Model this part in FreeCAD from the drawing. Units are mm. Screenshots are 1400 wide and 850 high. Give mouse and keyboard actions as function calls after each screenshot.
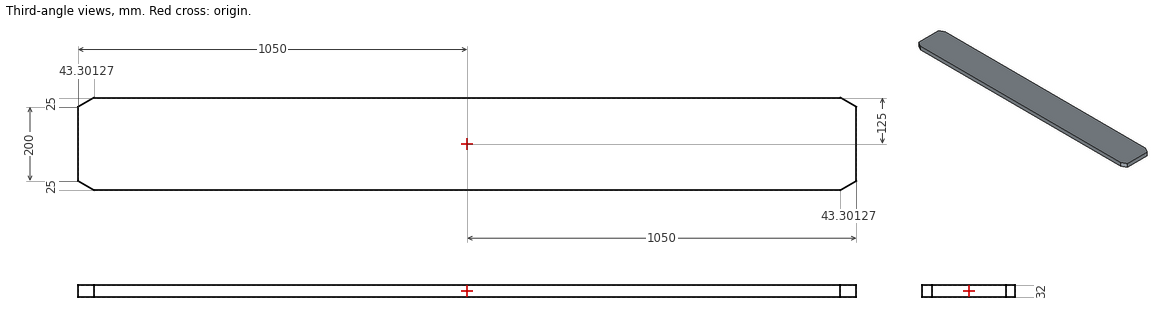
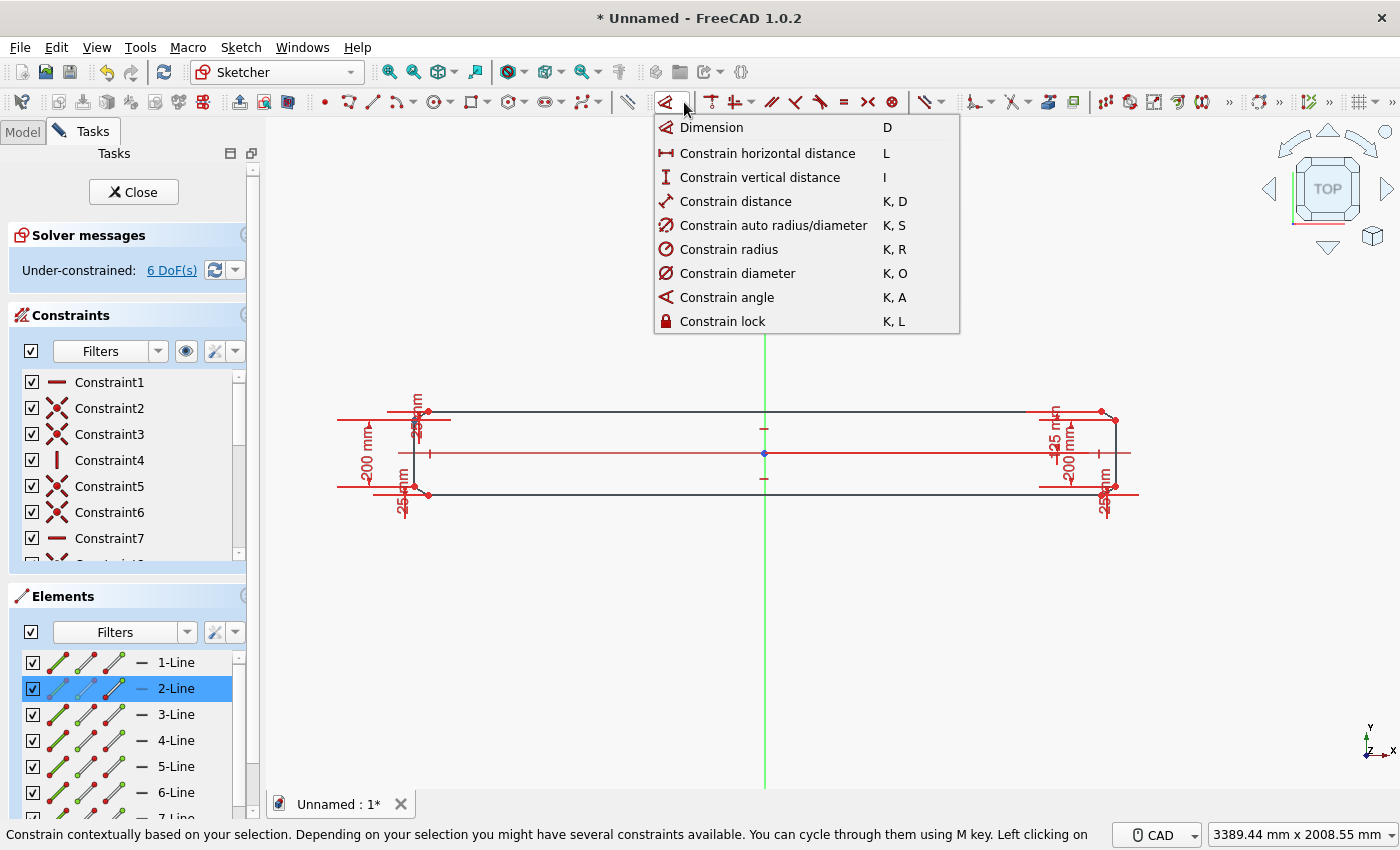
click(807, 153)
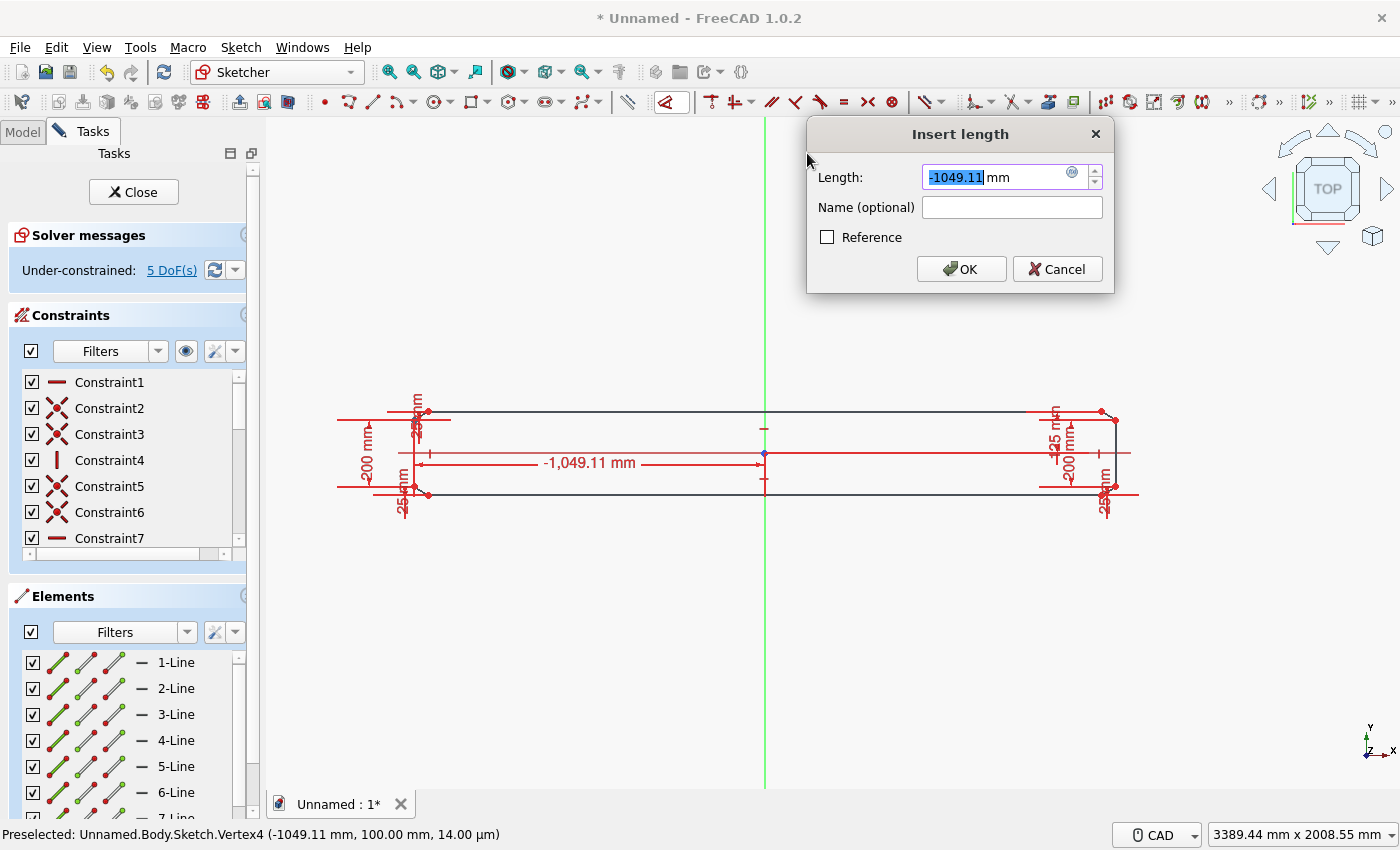
text(-1050)
key(Return)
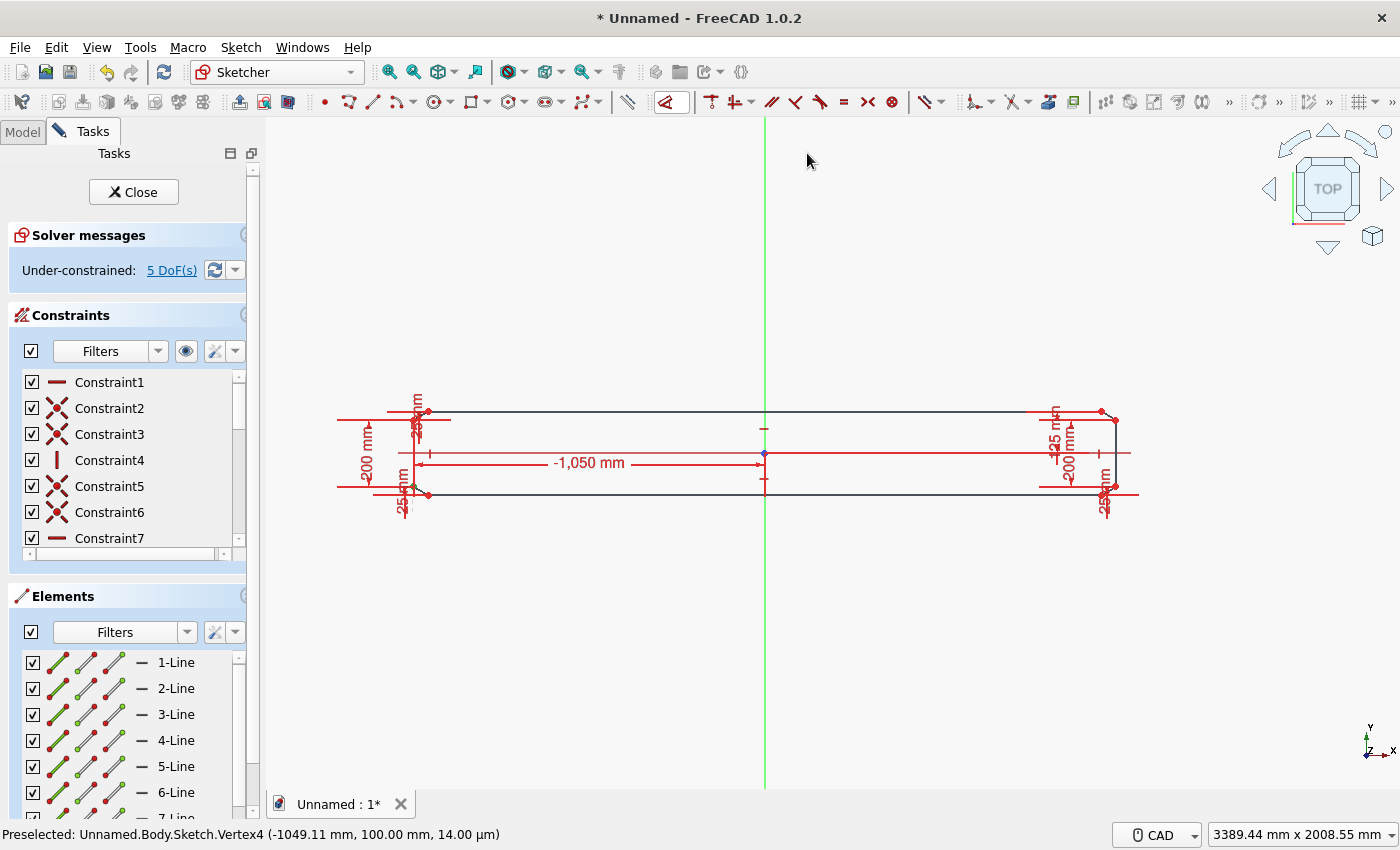
click(1116, 487)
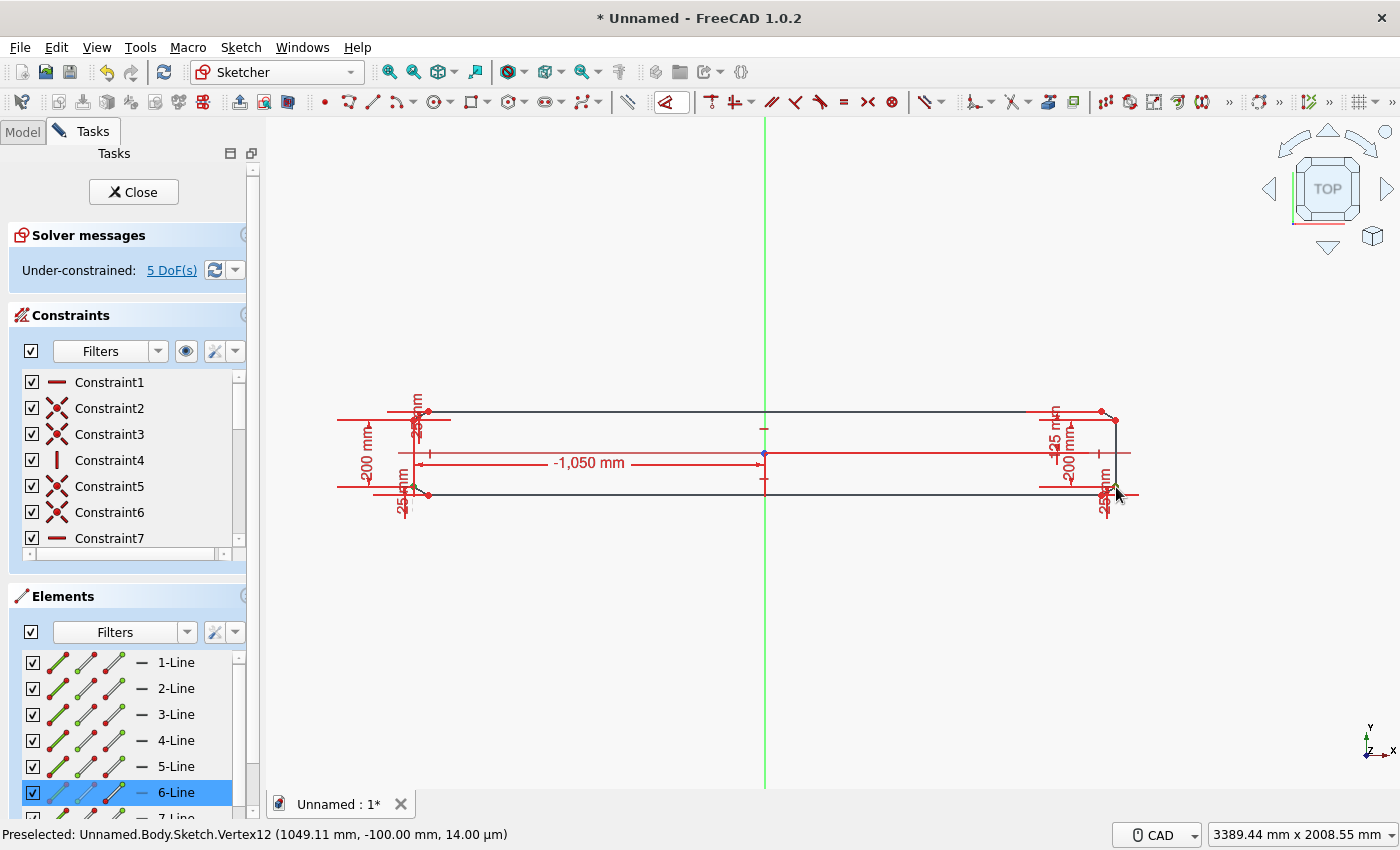
click(684, 102)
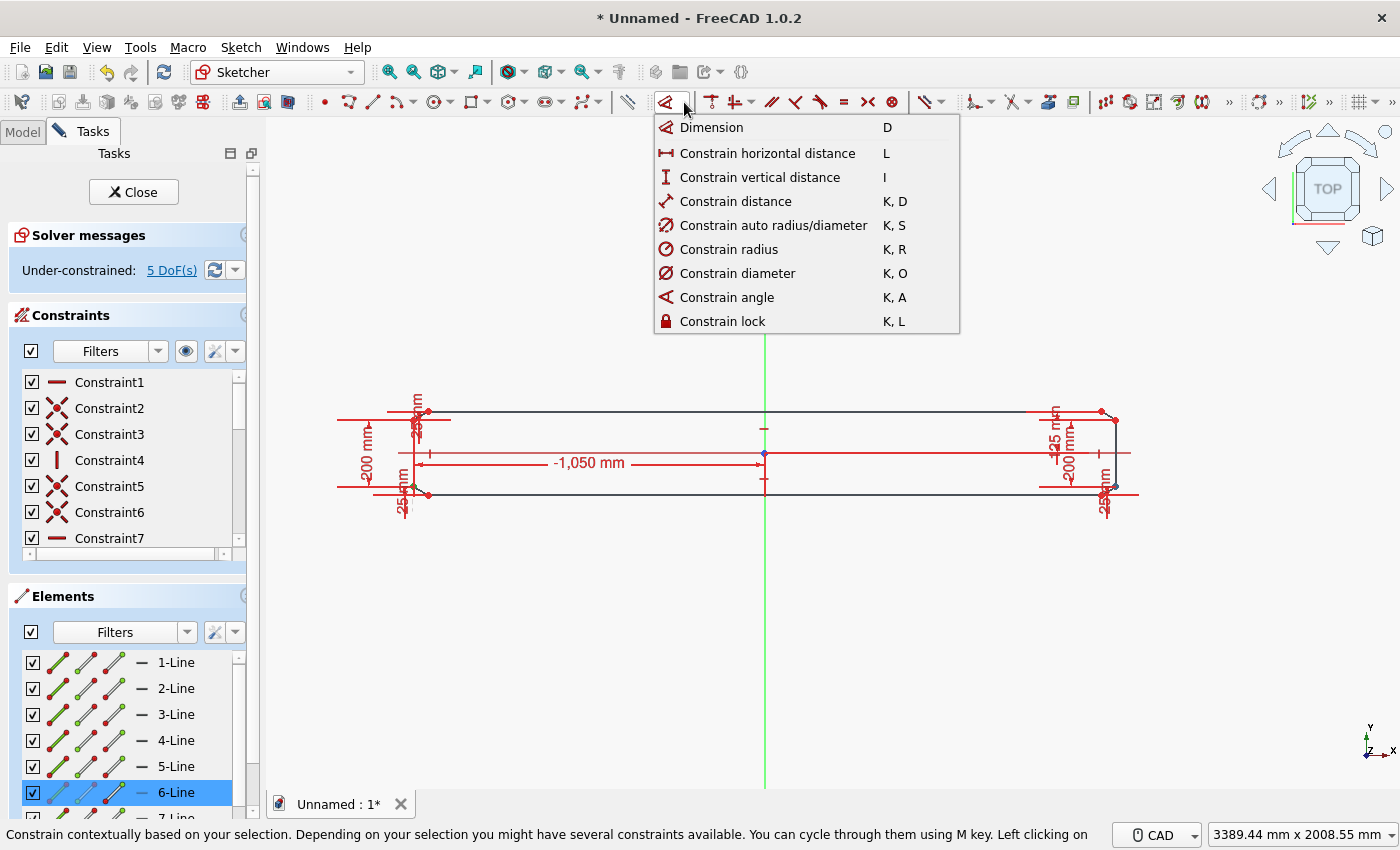
click(807, 153)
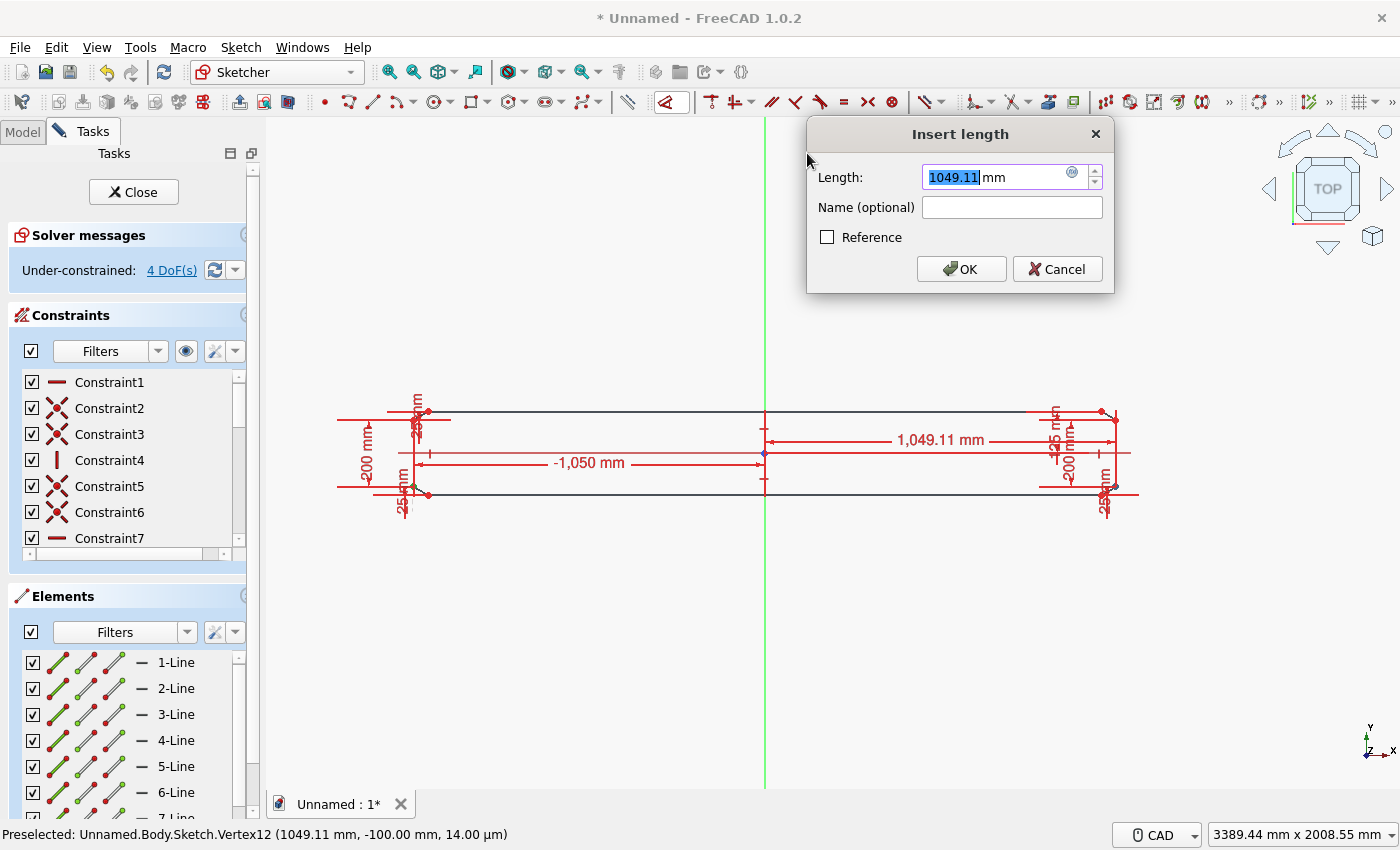
text(1050)
key(Return)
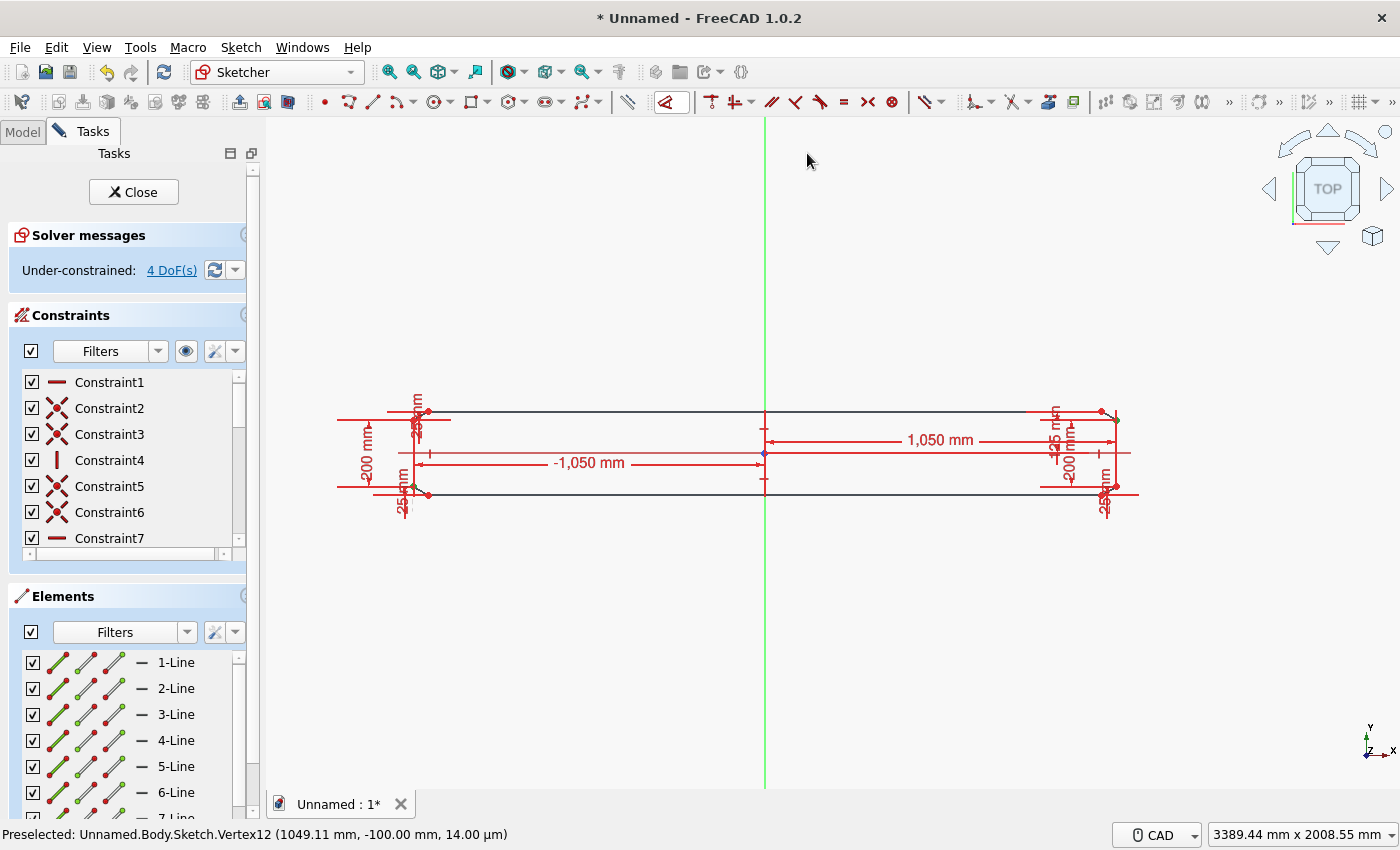
scroll(421, 416, up, 6)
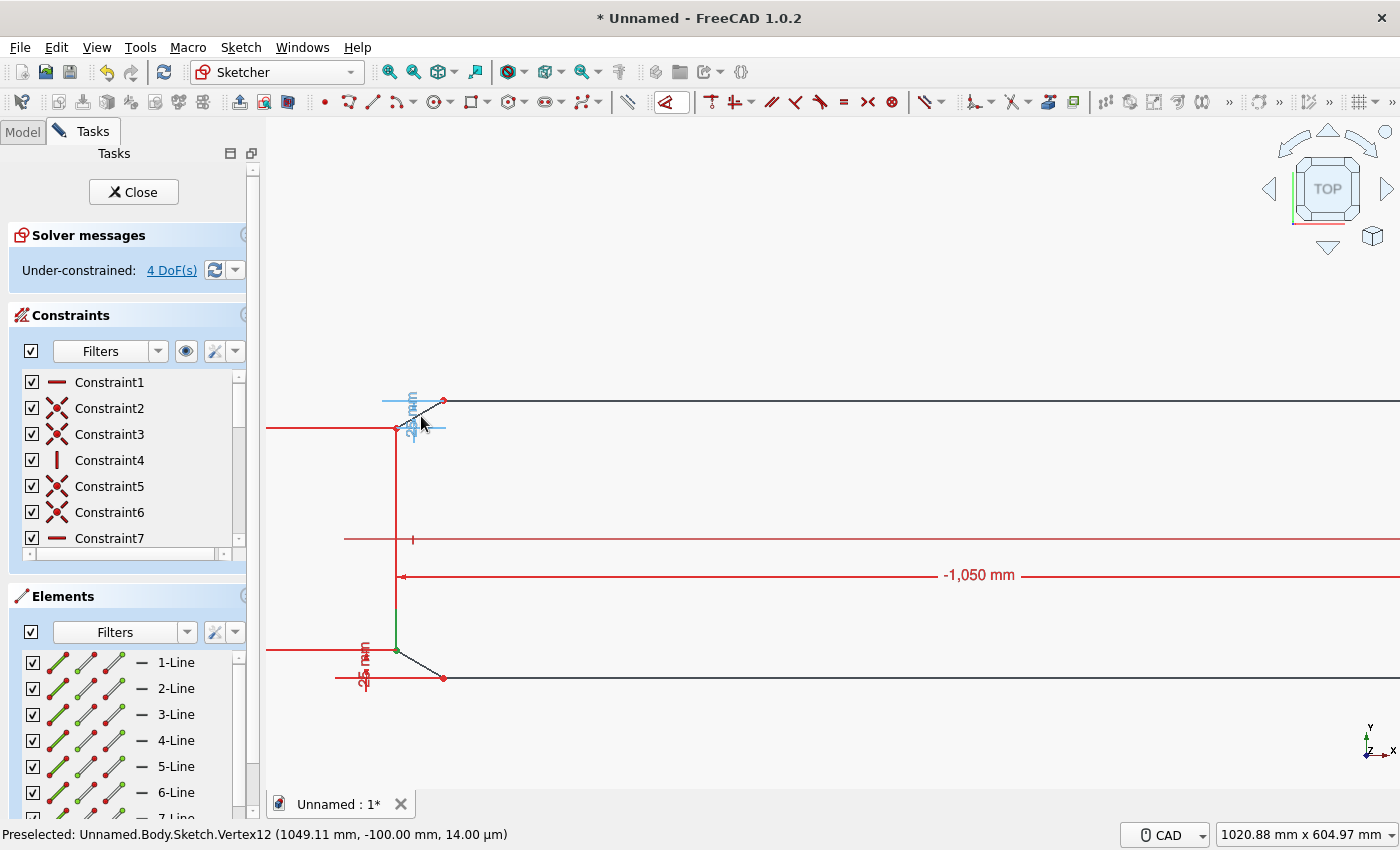
click(425, 412)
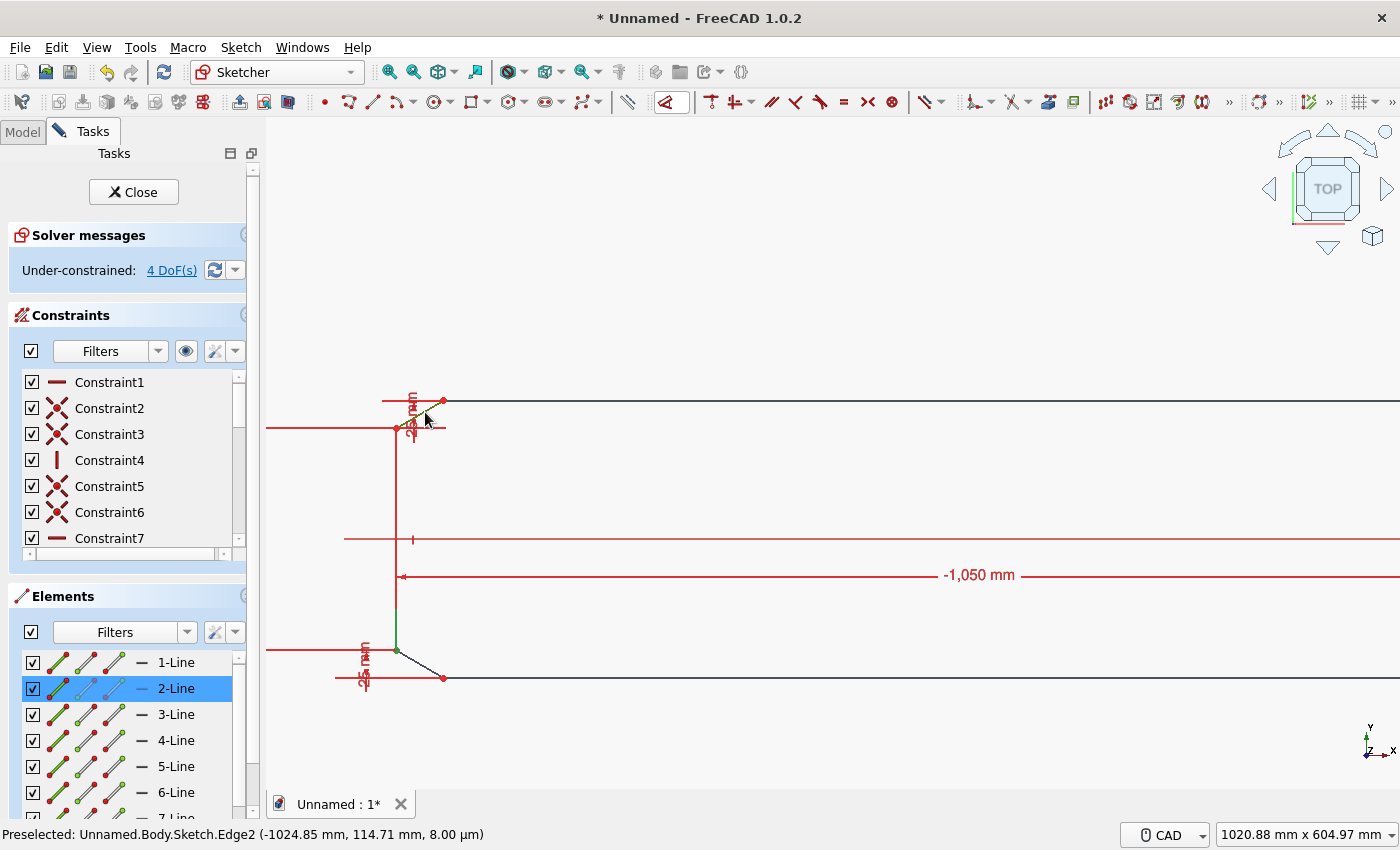
click(684, 102)